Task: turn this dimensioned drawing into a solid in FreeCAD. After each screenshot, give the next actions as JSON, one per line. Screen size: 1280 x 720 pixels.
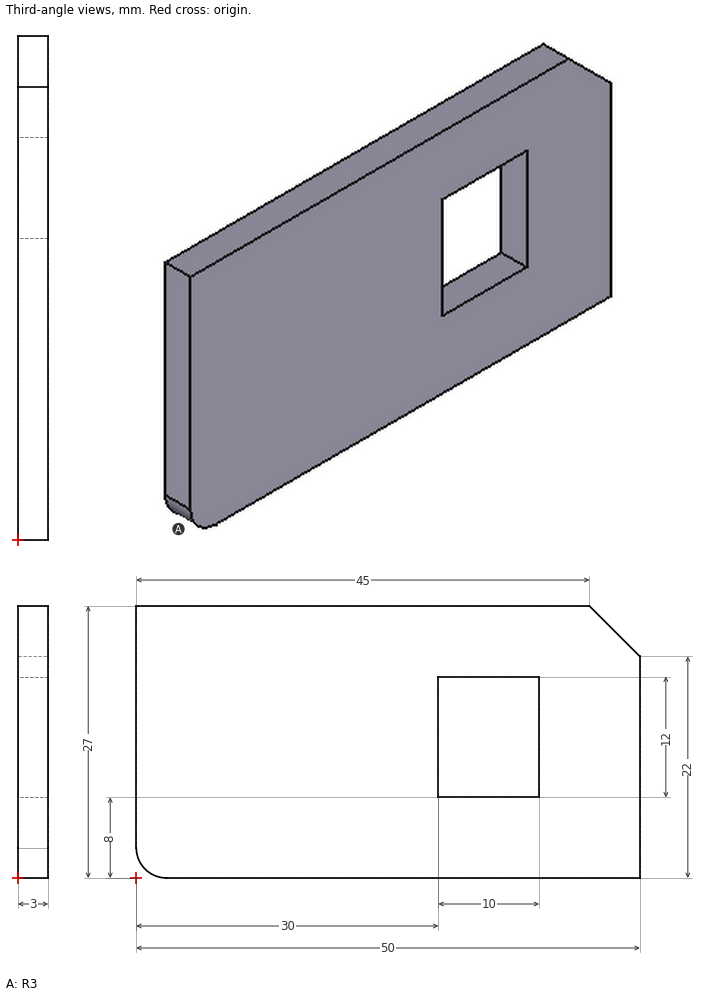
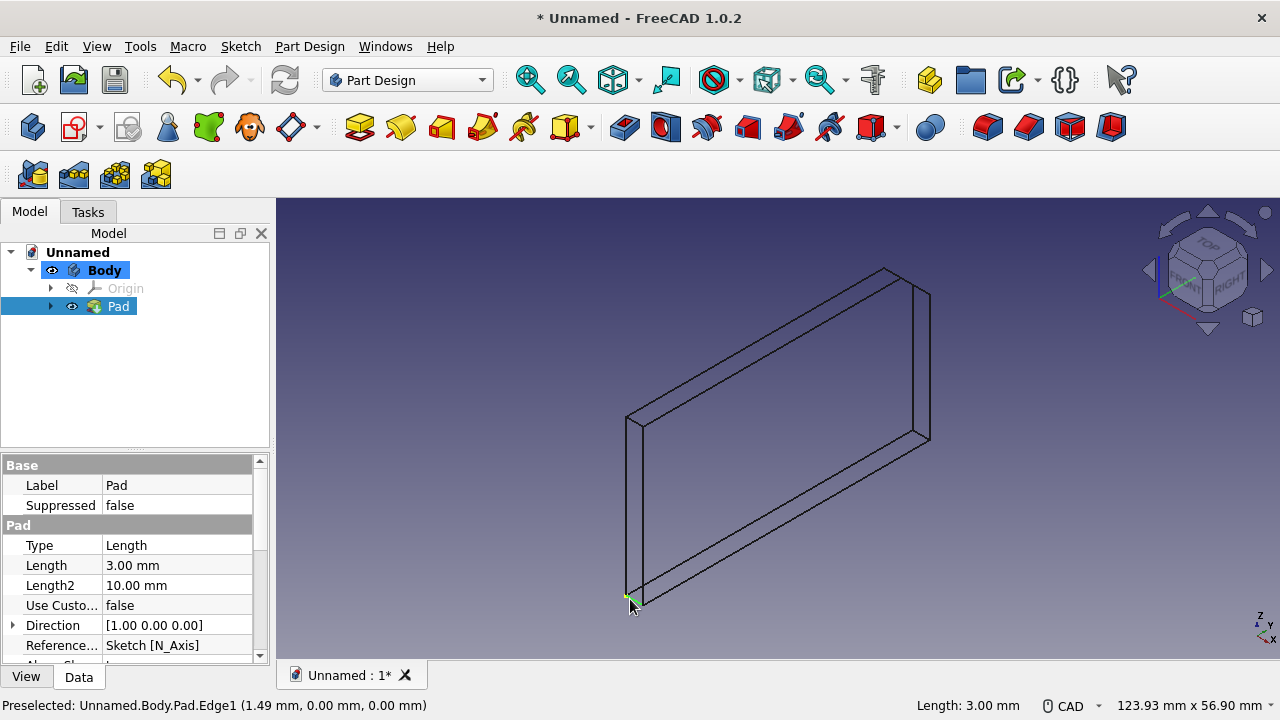
{"action": "left_click", "coordinate": [988, 128]}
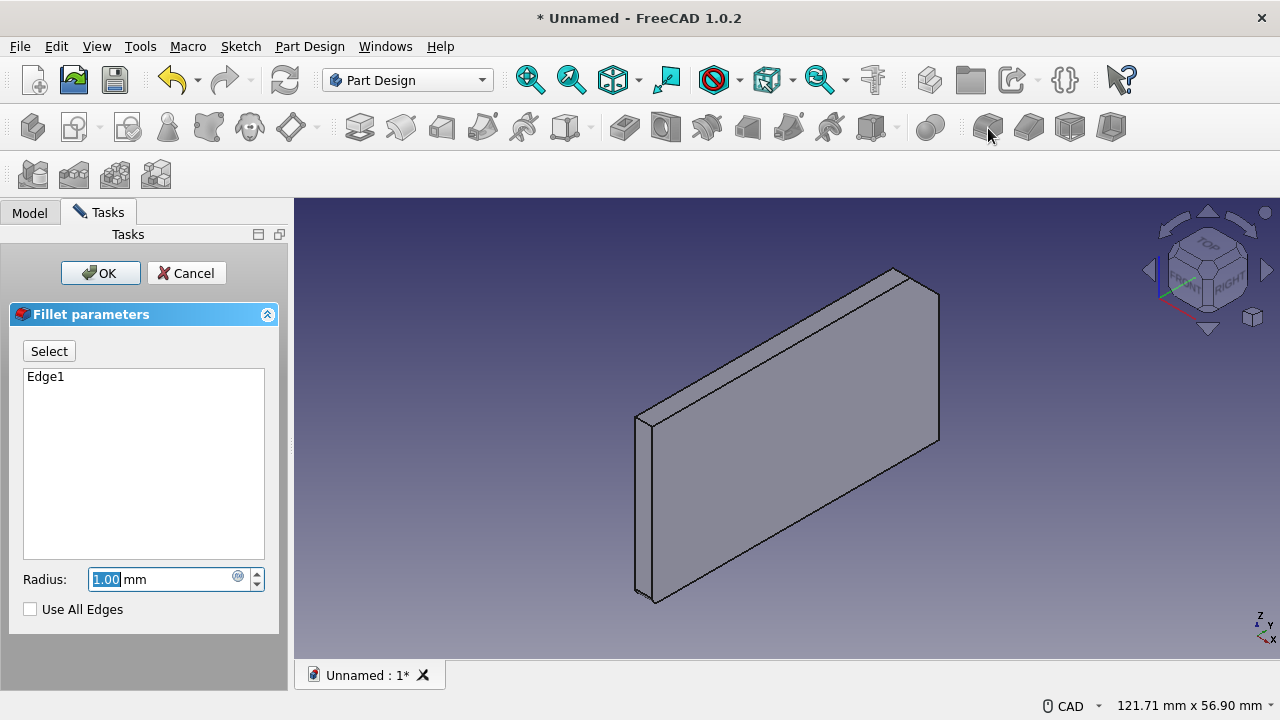
{"action": "type", "text": "3"}
{"action": "key", "text": "Tab"}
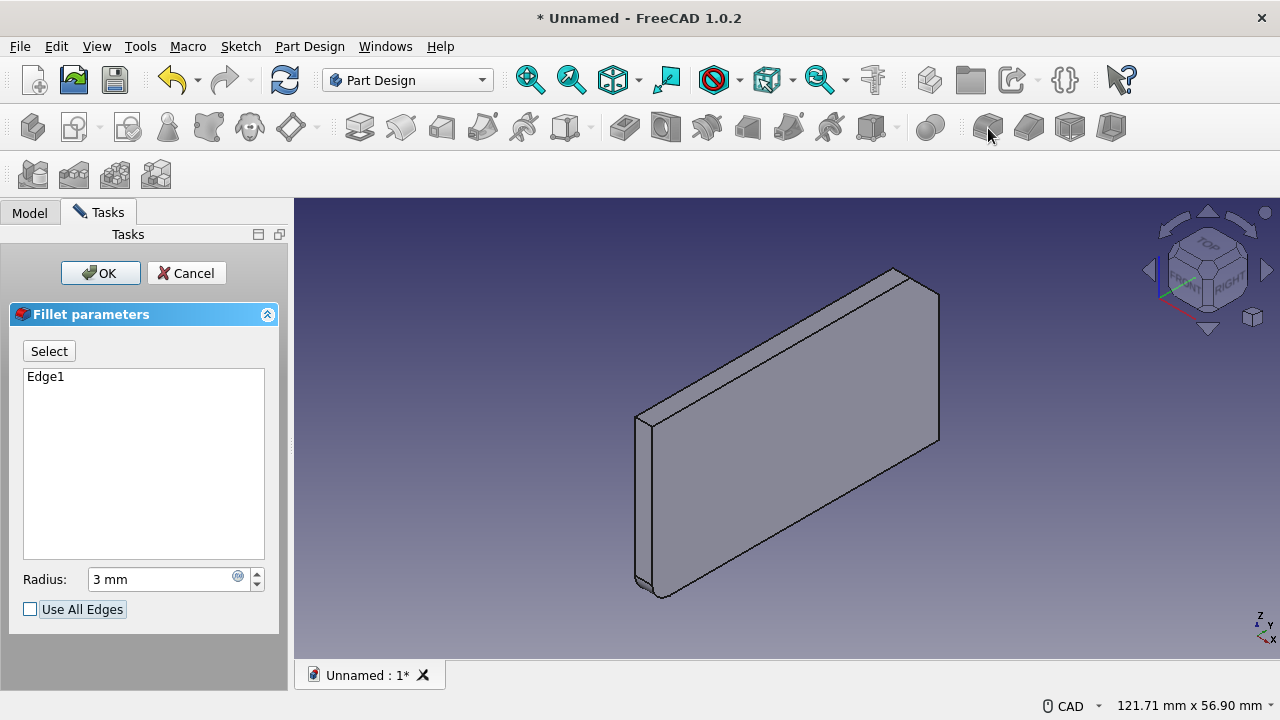
{"action": "left_click", "coordinate": [101, 273]}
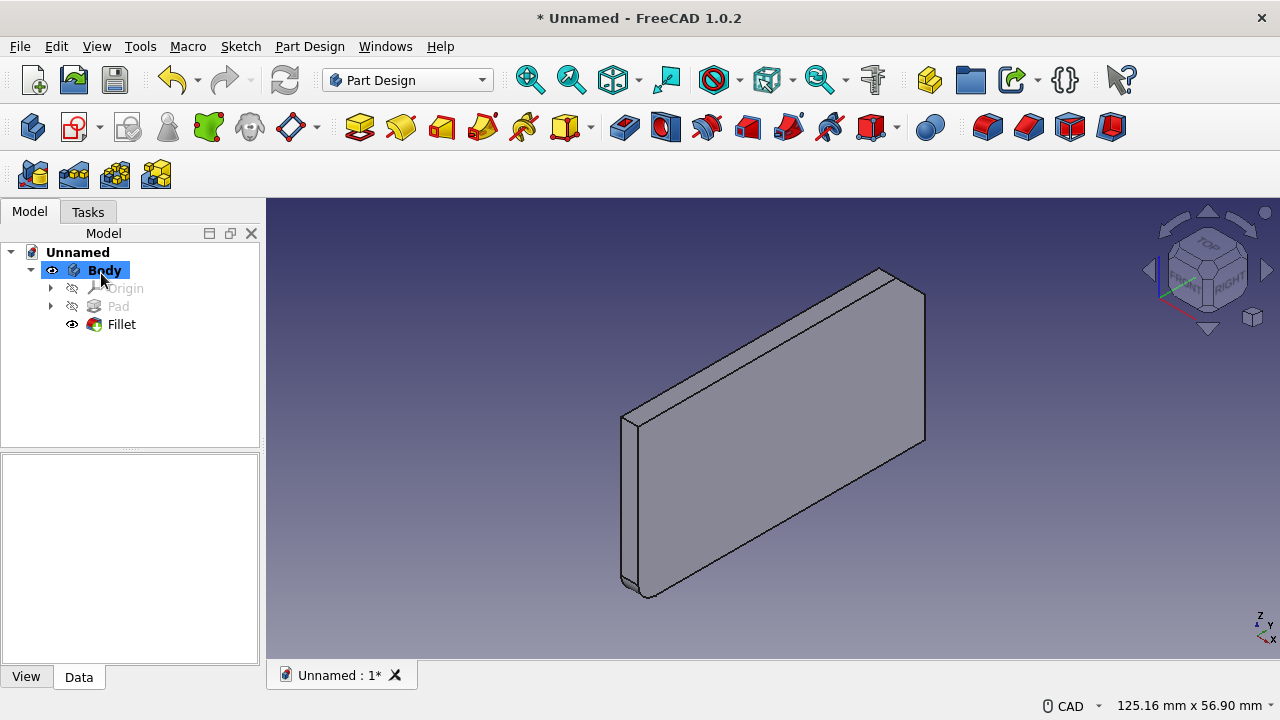
{"action": "left_click", "coordinate": [823, 409]}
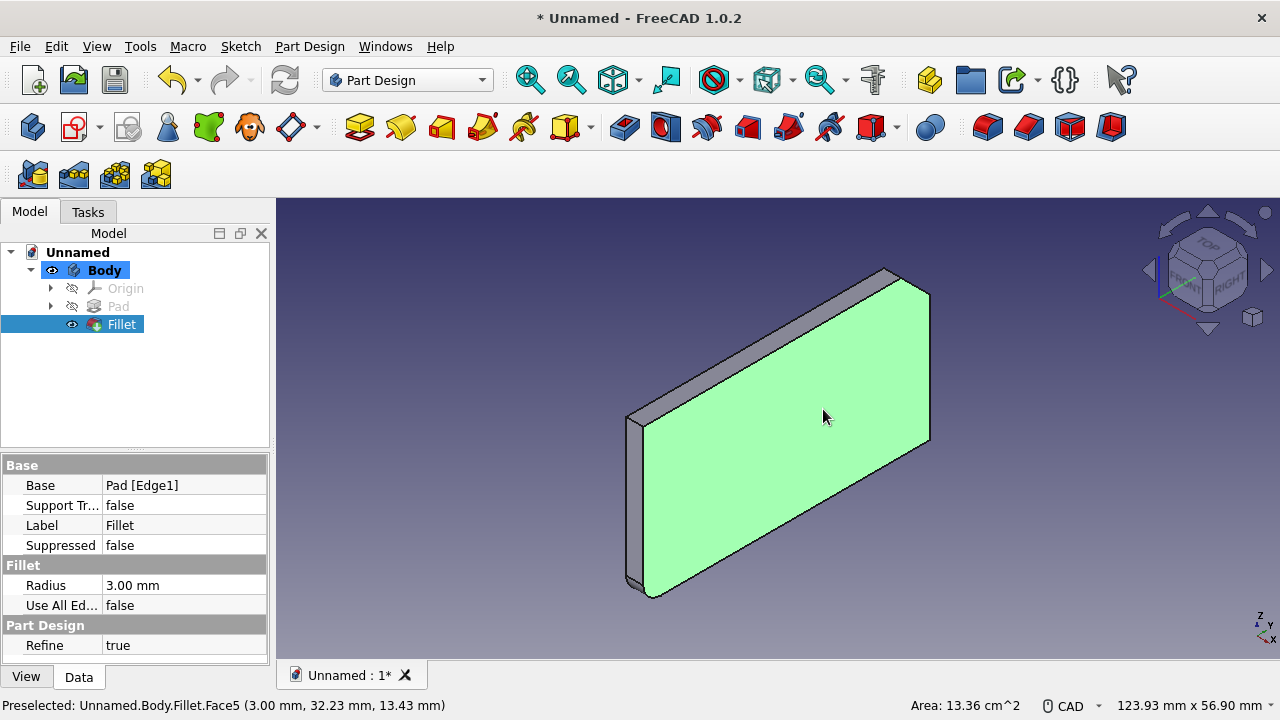
{"action": "left_click", "coordinate": [74, 128]}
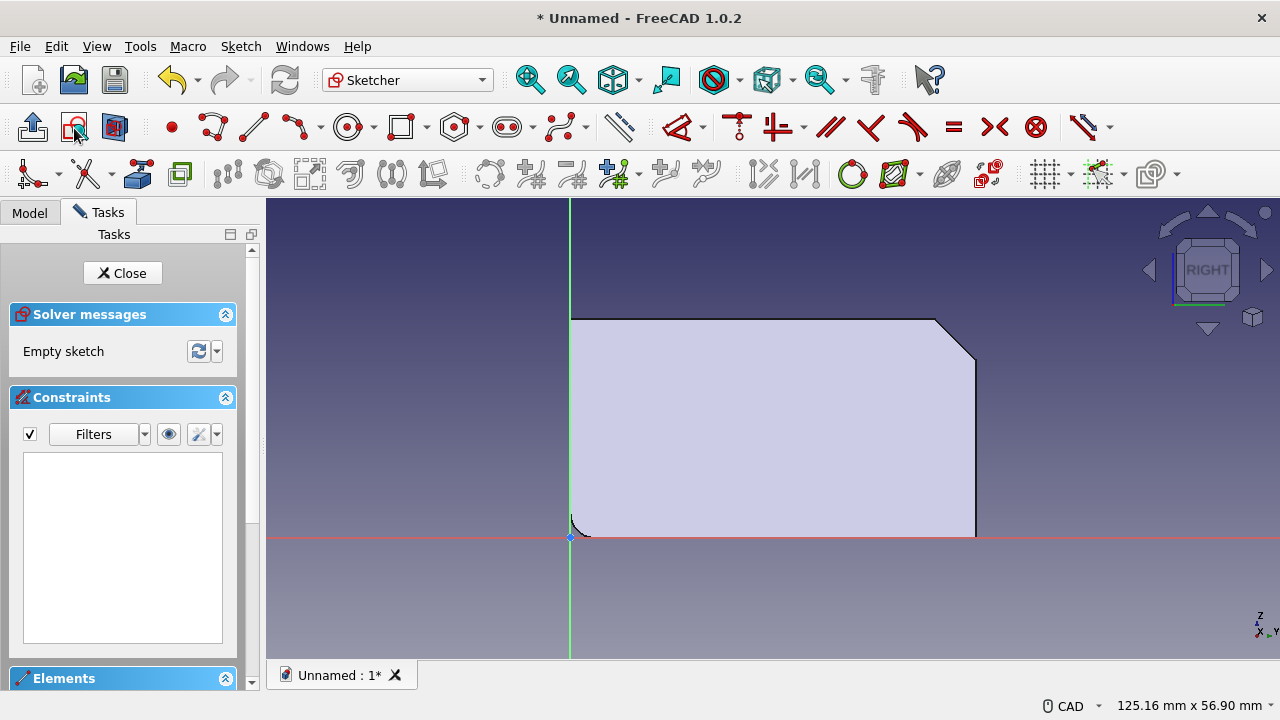
{"action": "scroll", "coordinate": [941, 422], "scroll_direction": "up", "scroll_amount": 5}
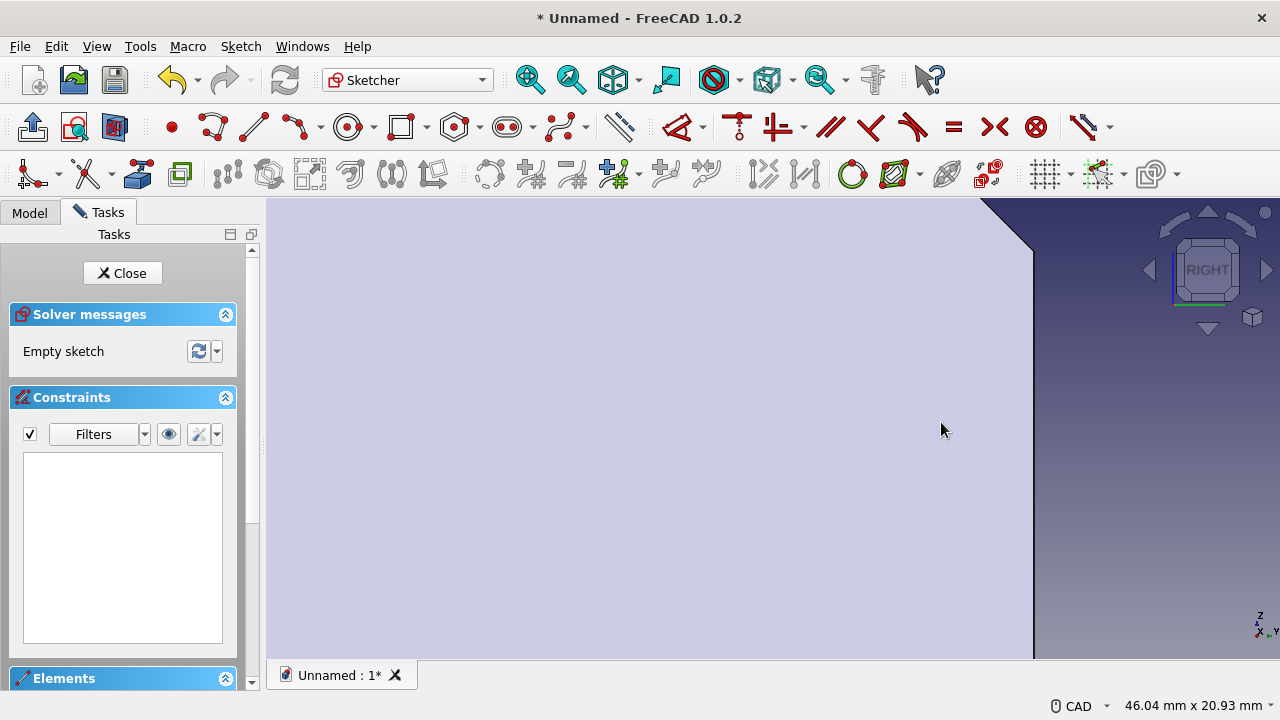
{"action": "key", "text": "g r"}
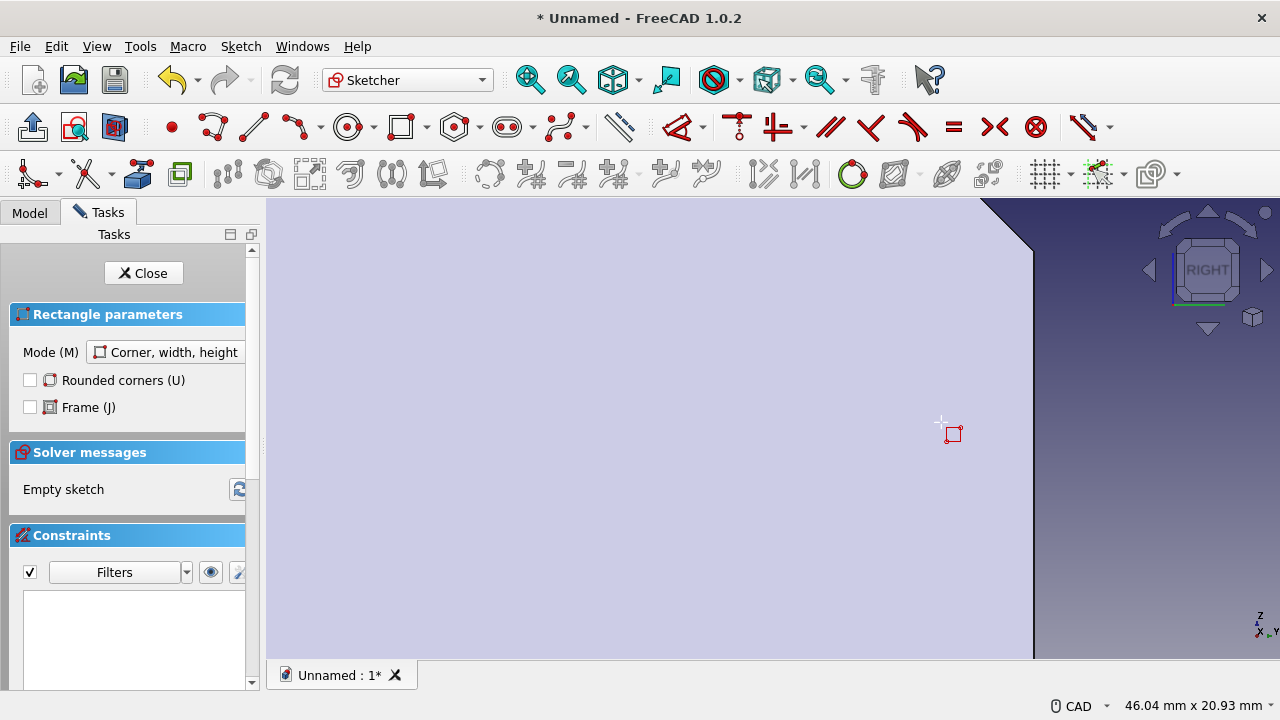
{"action": "left_click", "coordinate": [593, 296]}
{"action": "left_click", "coordinate": [814, 560]}
{"action": "key", "text": "Escape"}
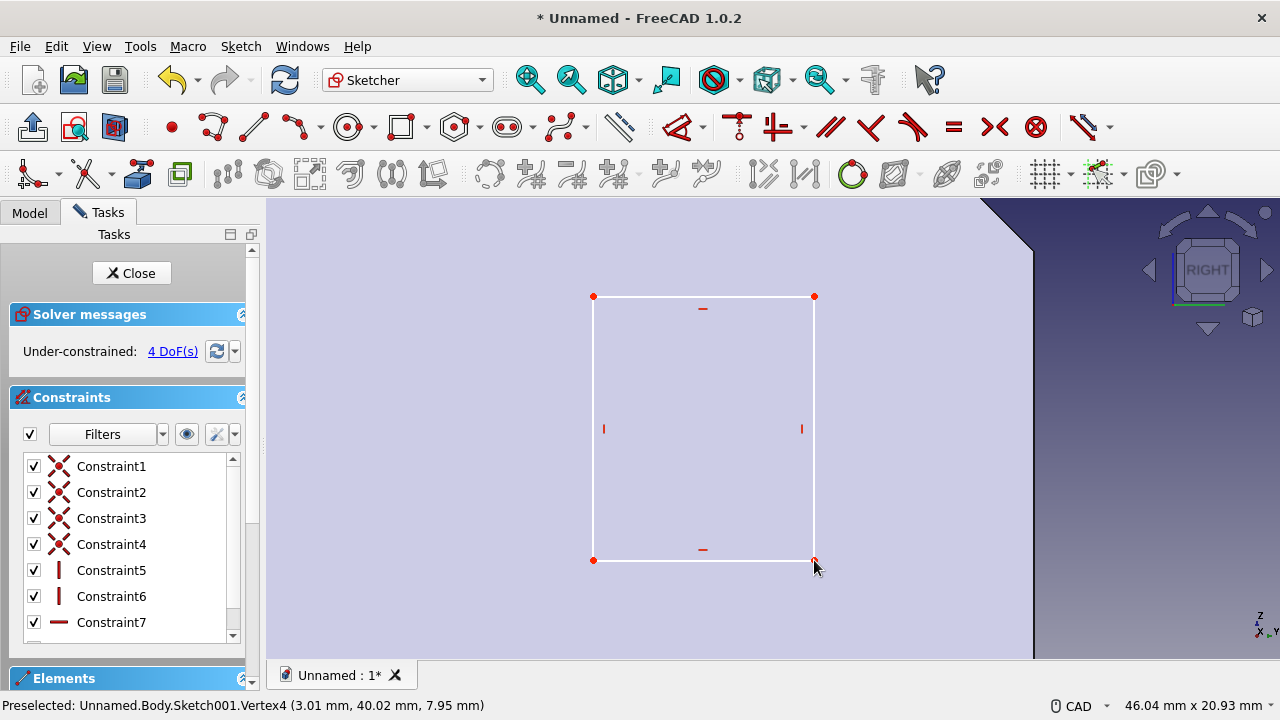
{"action": "left_click", "coordinate": [676, 128]}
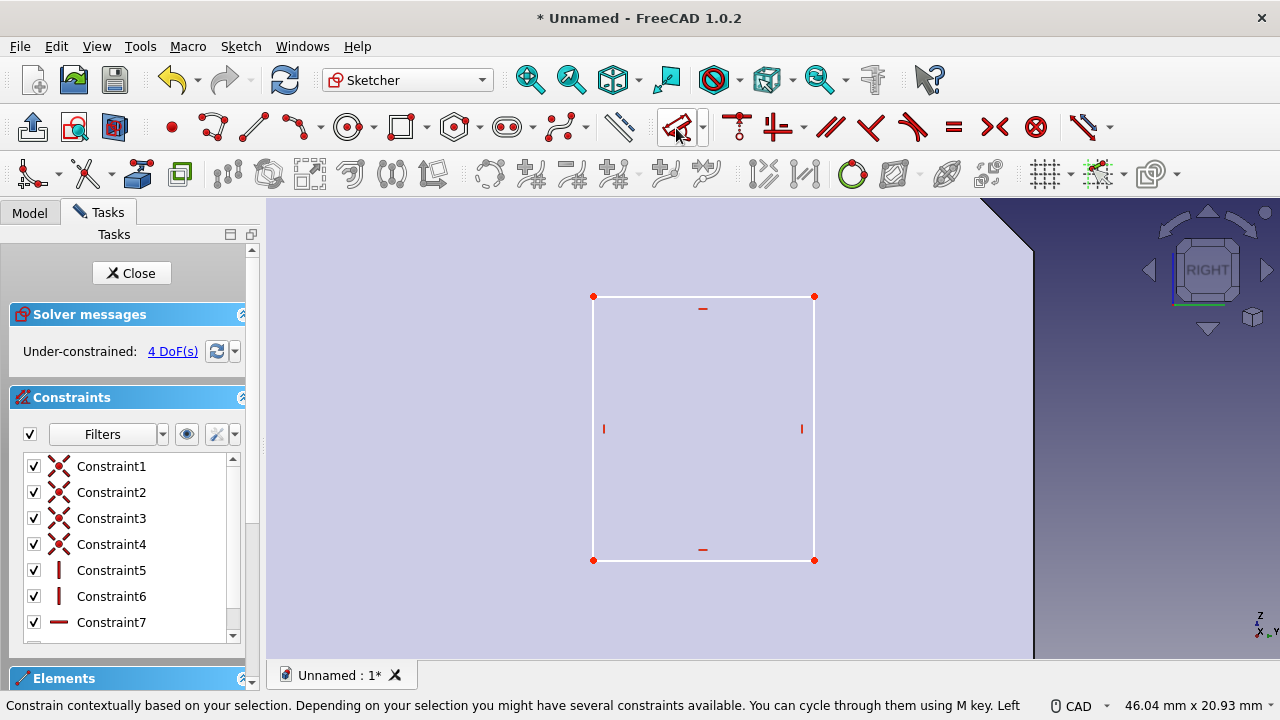
{"action": "left_click", "coordinate": [593, 376]}
{"action": "left_click", "coordinate": [559, 429]}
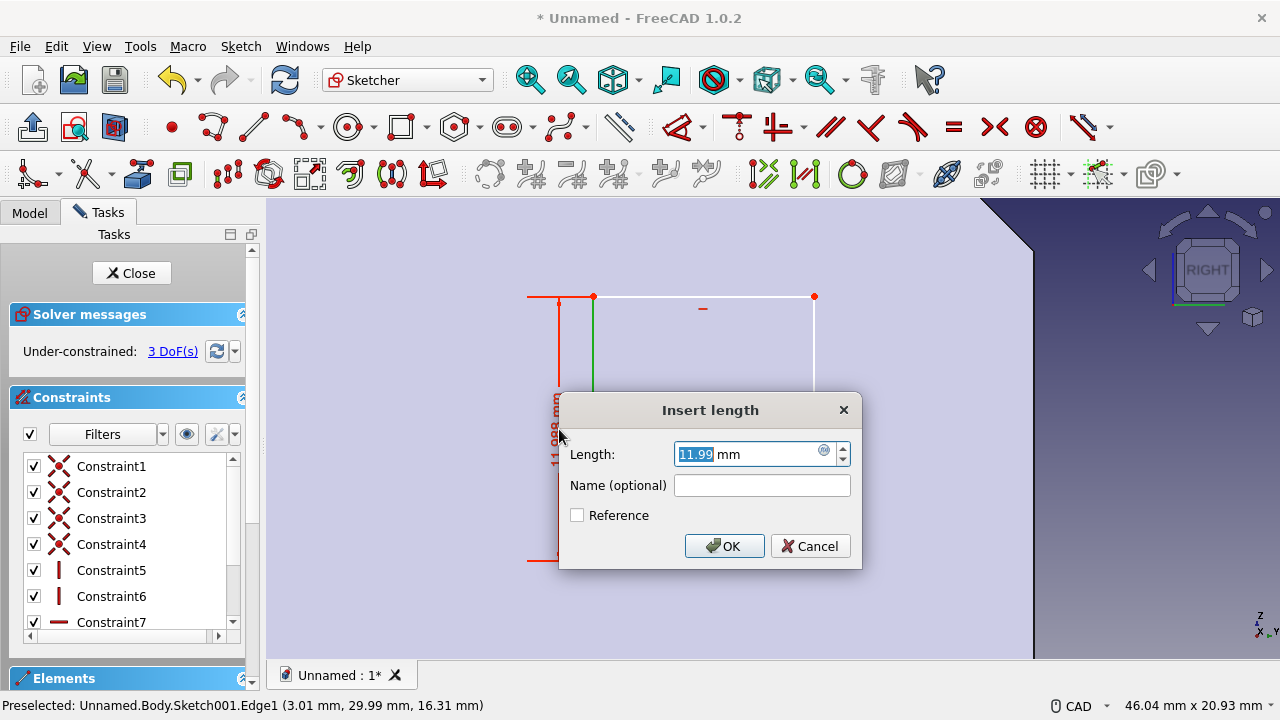
{"action": "type", "text": "12"}
{"action": "key", "text": "Return"}